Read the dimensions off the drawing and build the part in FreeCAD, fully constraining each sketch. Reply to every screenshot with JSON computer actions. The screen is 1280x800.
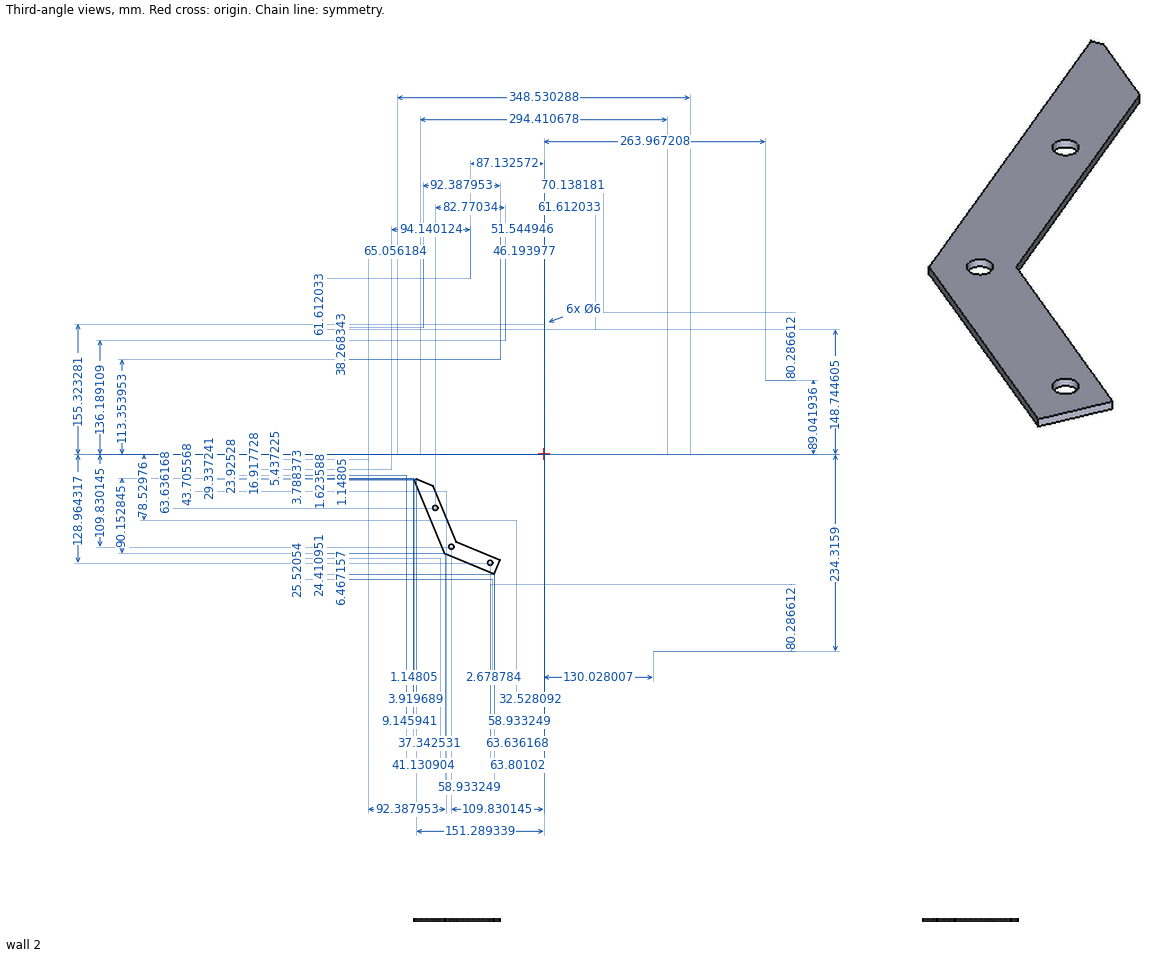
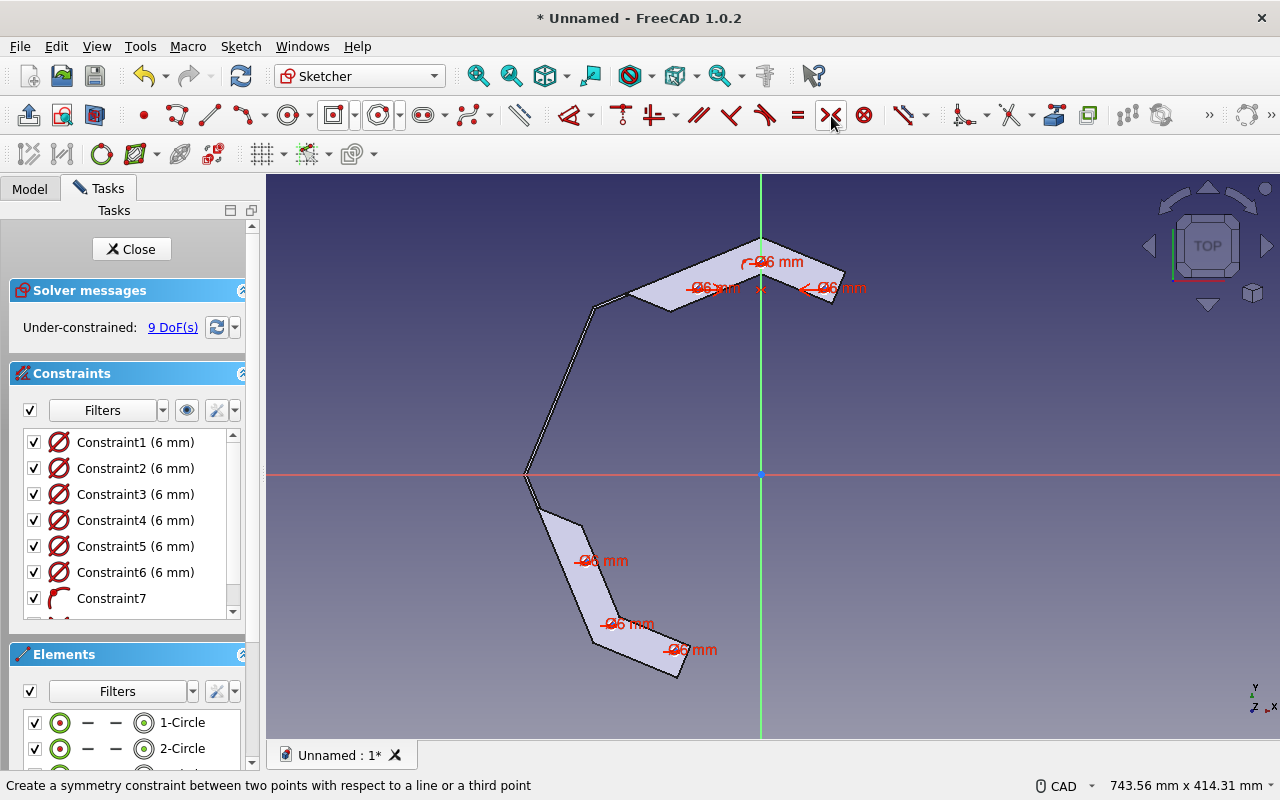
{"action": "left_click", "coordinate": [568, 116]}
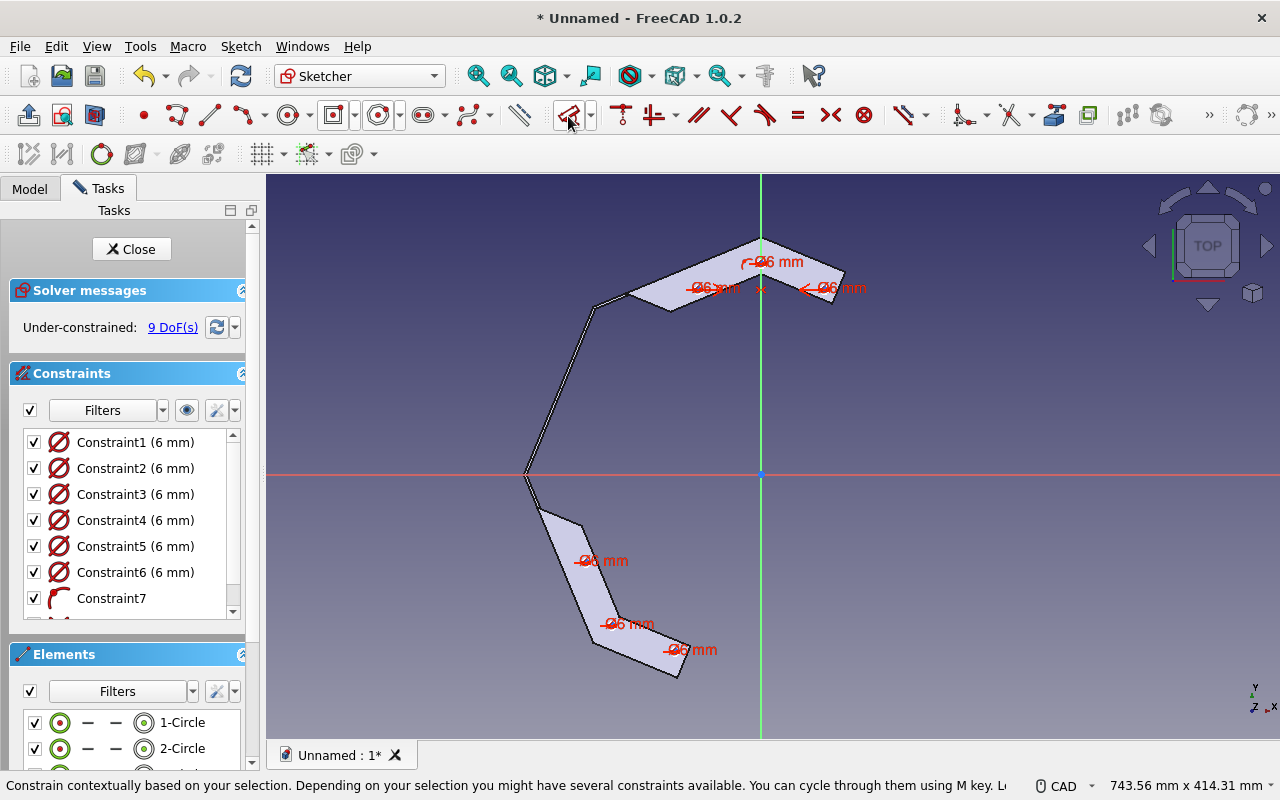
{"action": "left_click", "coordinate": [698, 290]}
{"action": "left_click", "coordinate": [730, 256]}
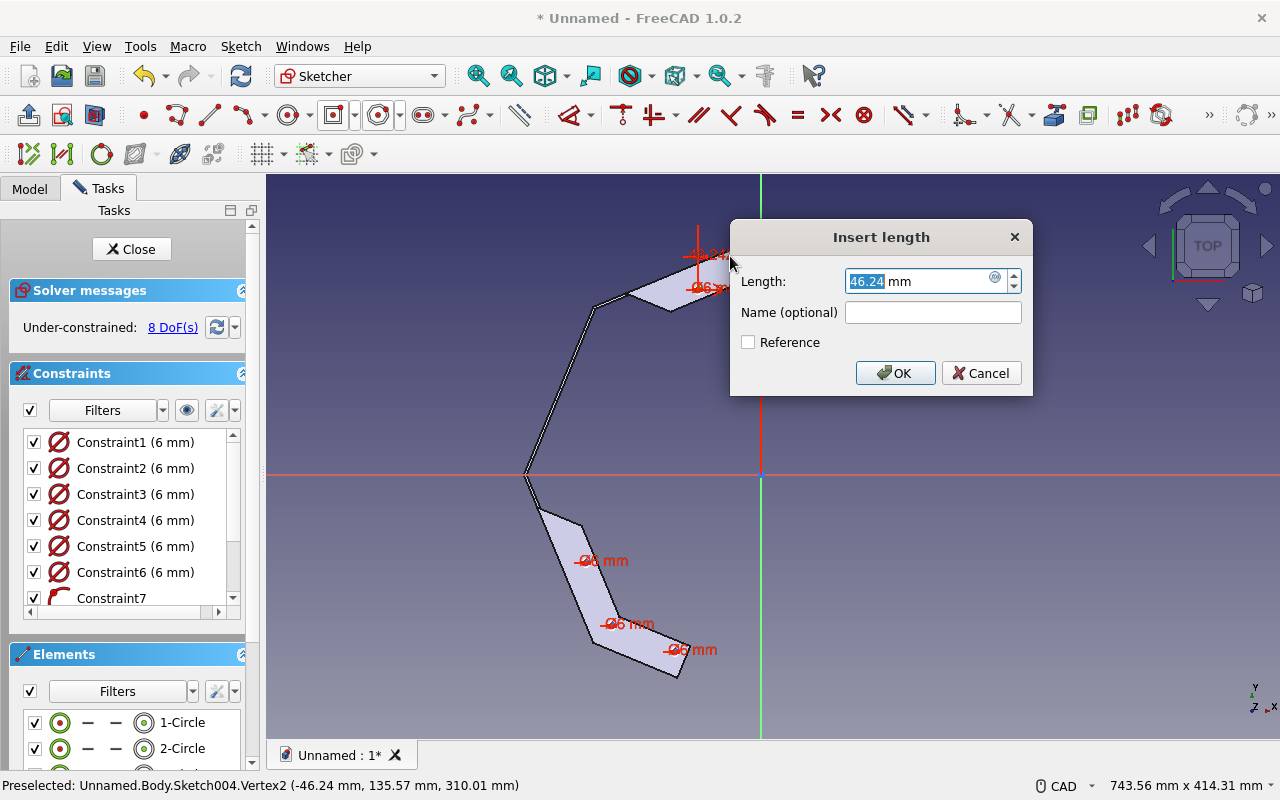
{"action": "type", "text": "46.193977"}
{"action": "key", "text": "Return"}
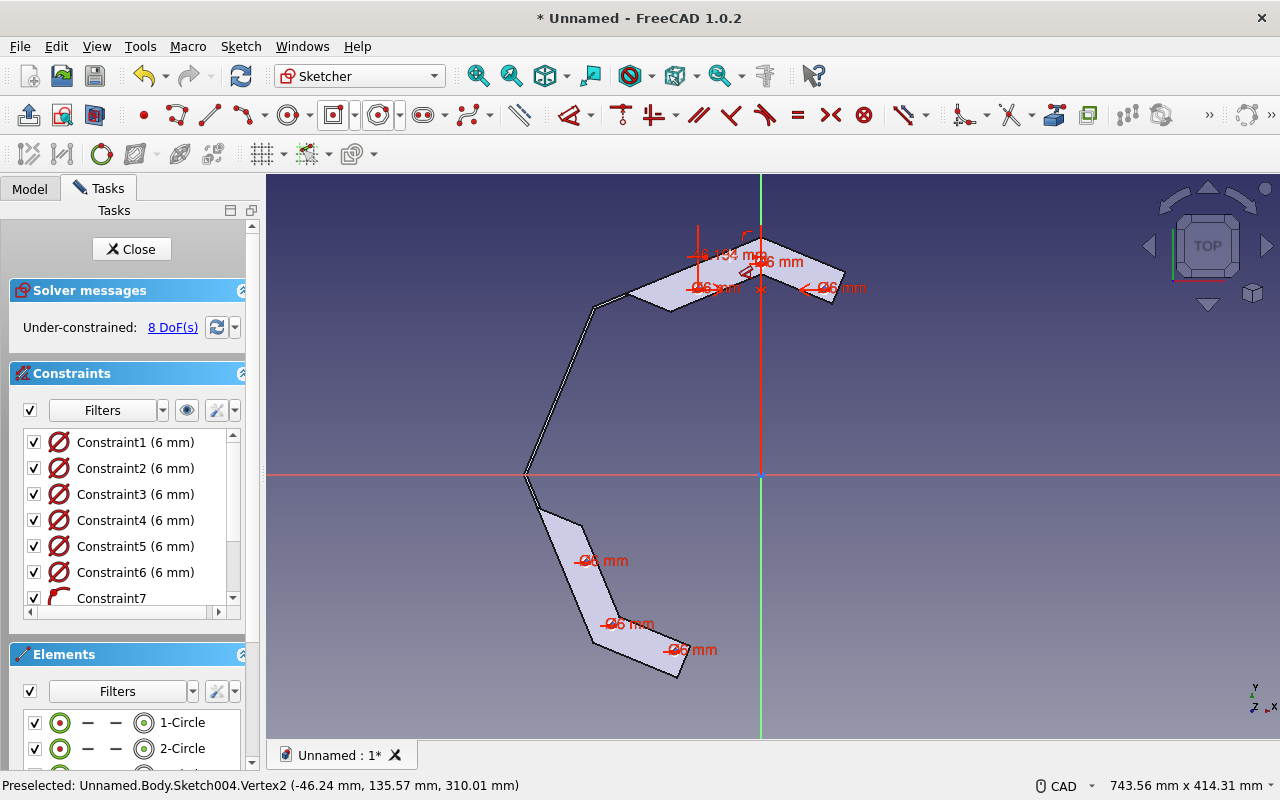
{"action": "left_click", "coordinate": [586, 563]}
{"action": "left_click", "coordinate": [552, 519]}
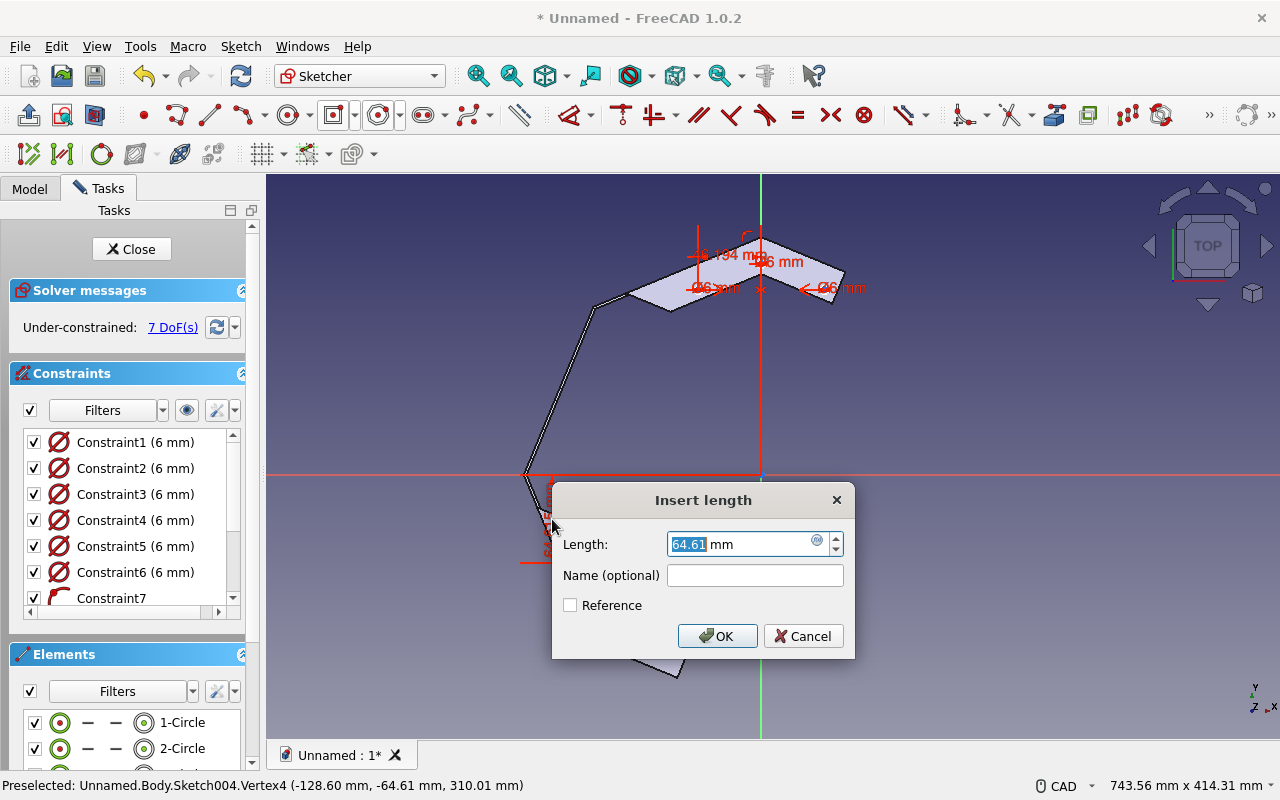
{"action": "type", "text": "63.636168"}
{"action": "key", "text": "Return"}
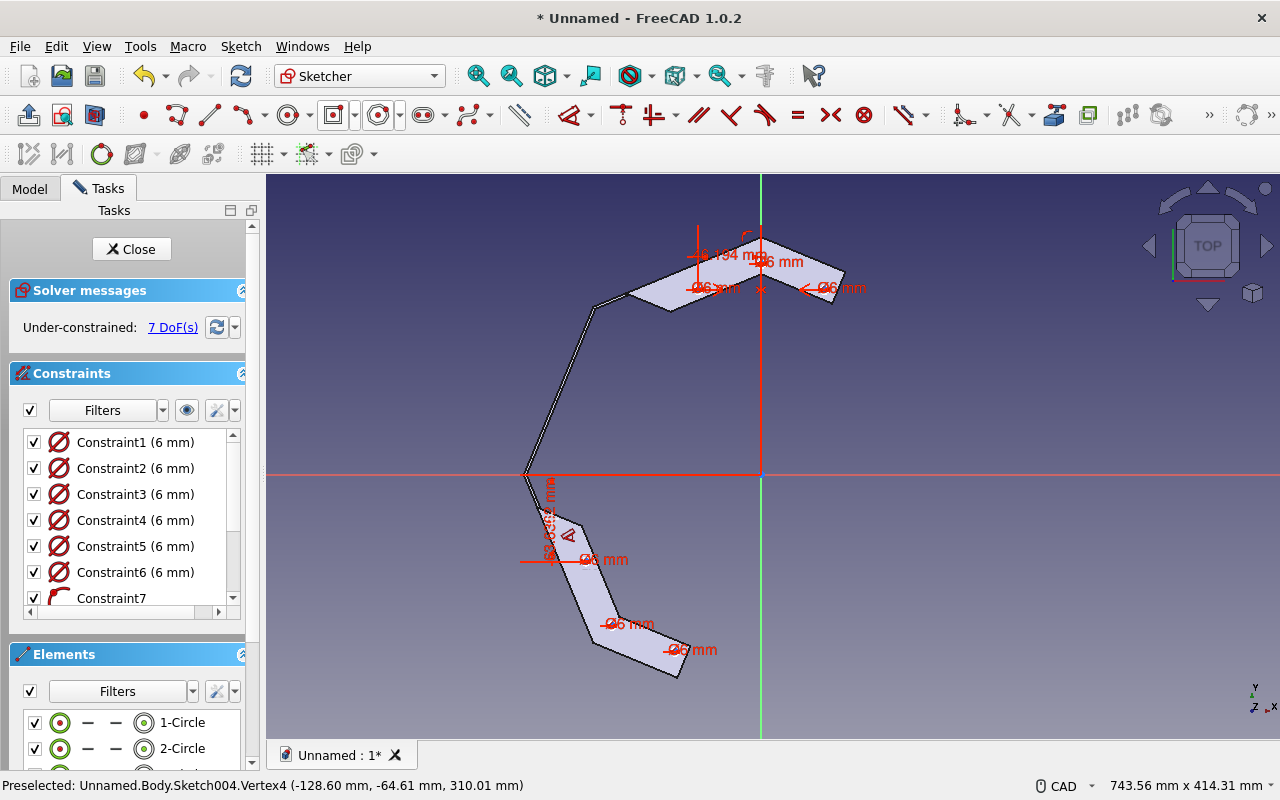
{"action": "left_click", "coordinate": [675, 652]}
{"action": "left_click", "coordinate": [718, 686]}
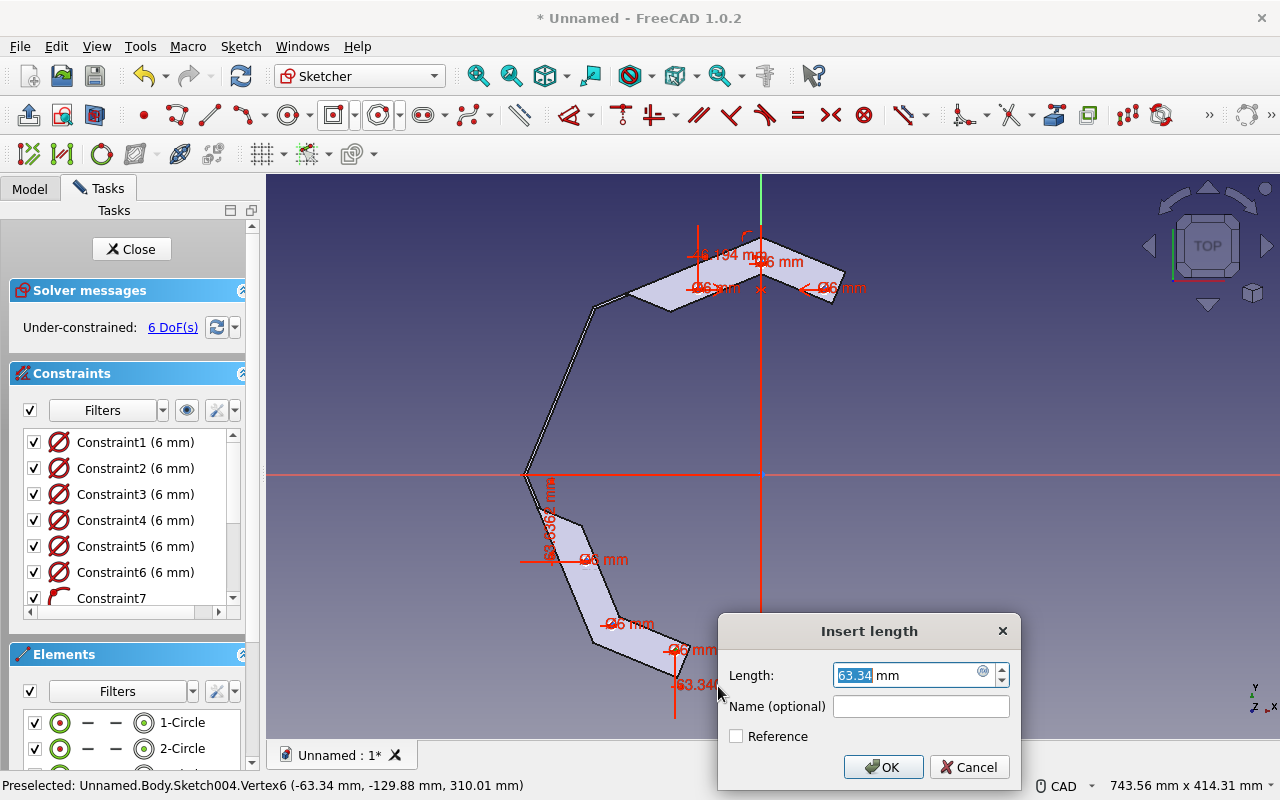
{"action": "type", "text": "63.636168"}
{"action": "key", "text": "Return"}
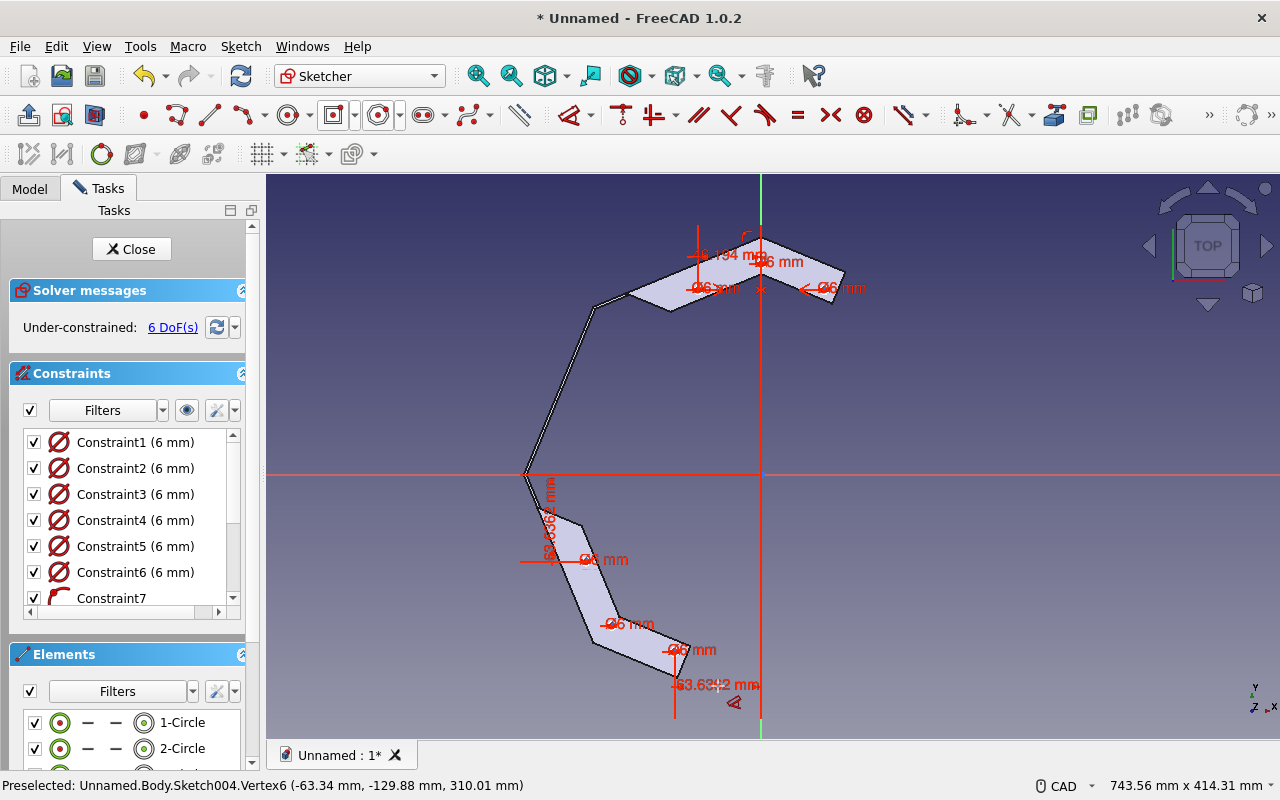
{"action": "left_click", "coordinate": [698, 290]}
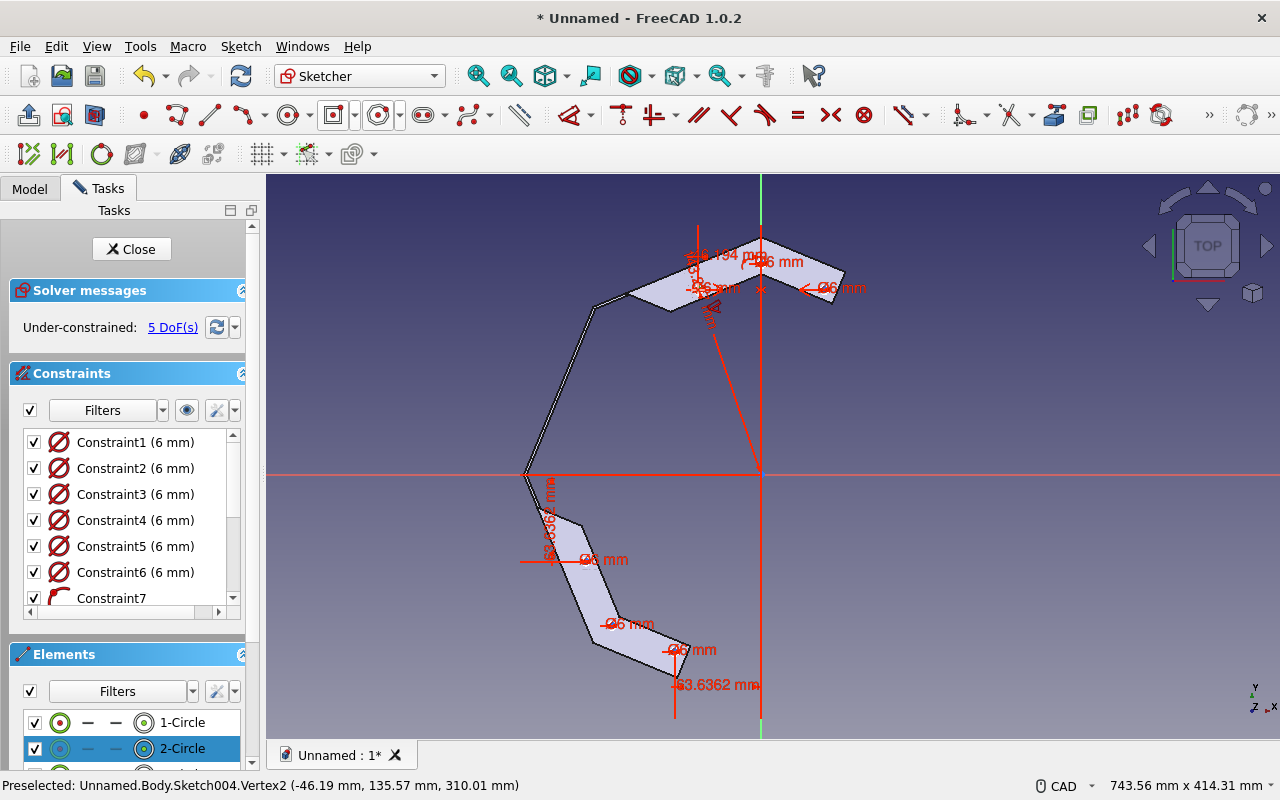
{"action": "left_click", "coordinate": [586, 562]}
{"action": "left_click", "coordinate": [642, 256]}